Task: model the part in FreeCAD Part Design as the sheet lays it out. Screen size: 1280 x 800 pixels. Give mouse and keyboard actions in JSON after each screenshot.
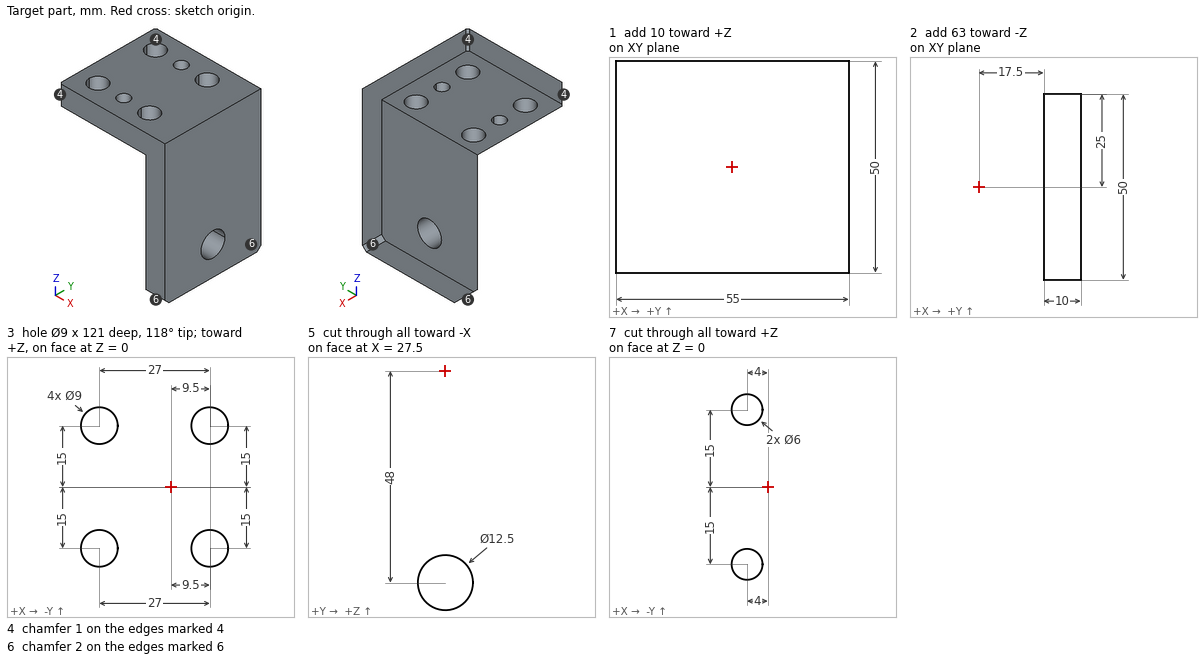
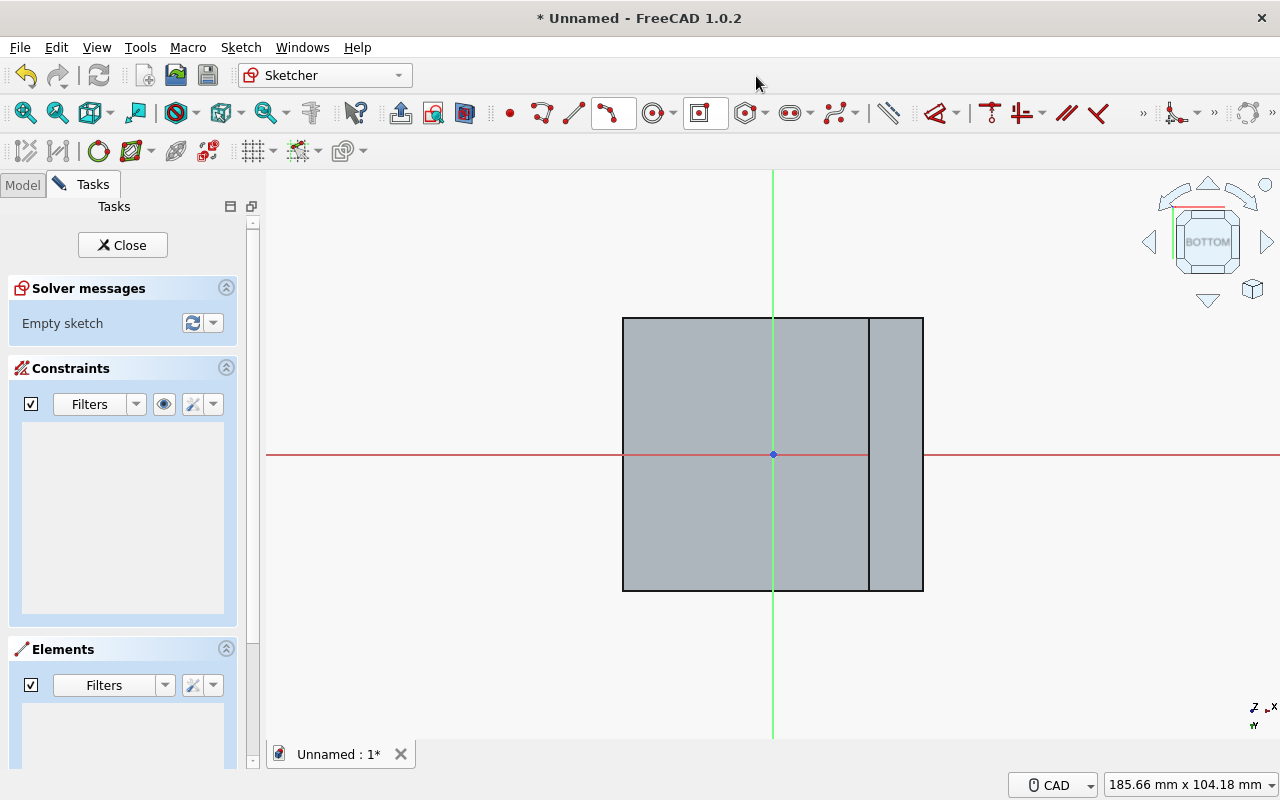
{"action": "left_click", "coordinate": [466, 114]}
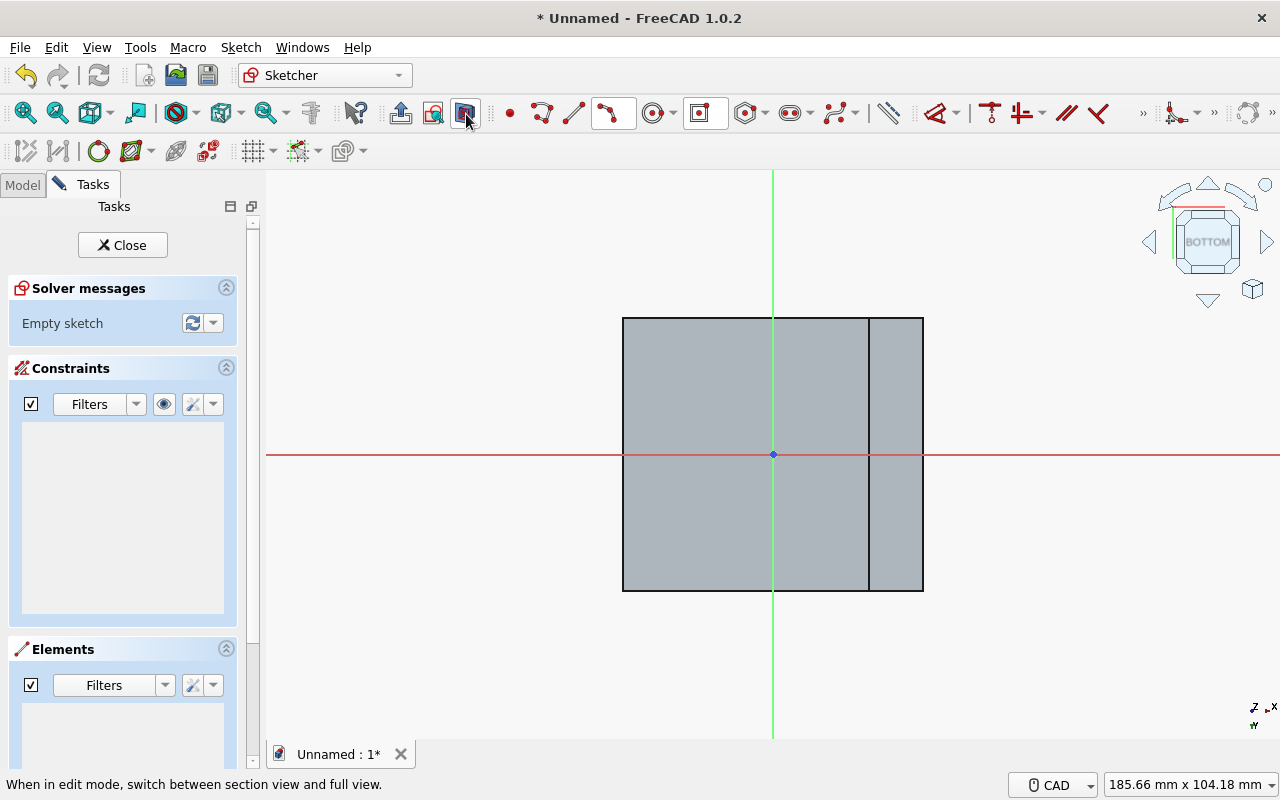
{"action": "scroll", "coordinate": [808, 454], "scroll_direction": "up", "scroll_amount": 3}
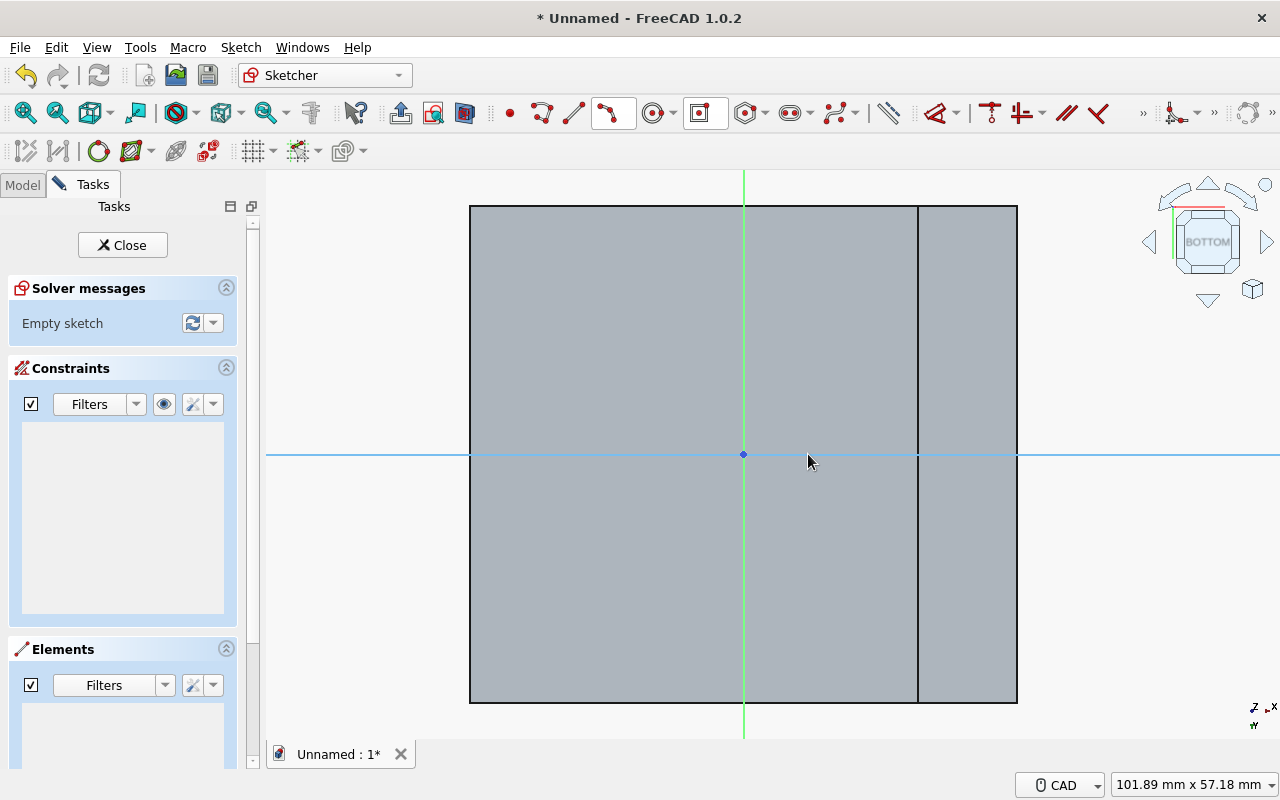
{"action": "key", "text": "g c"}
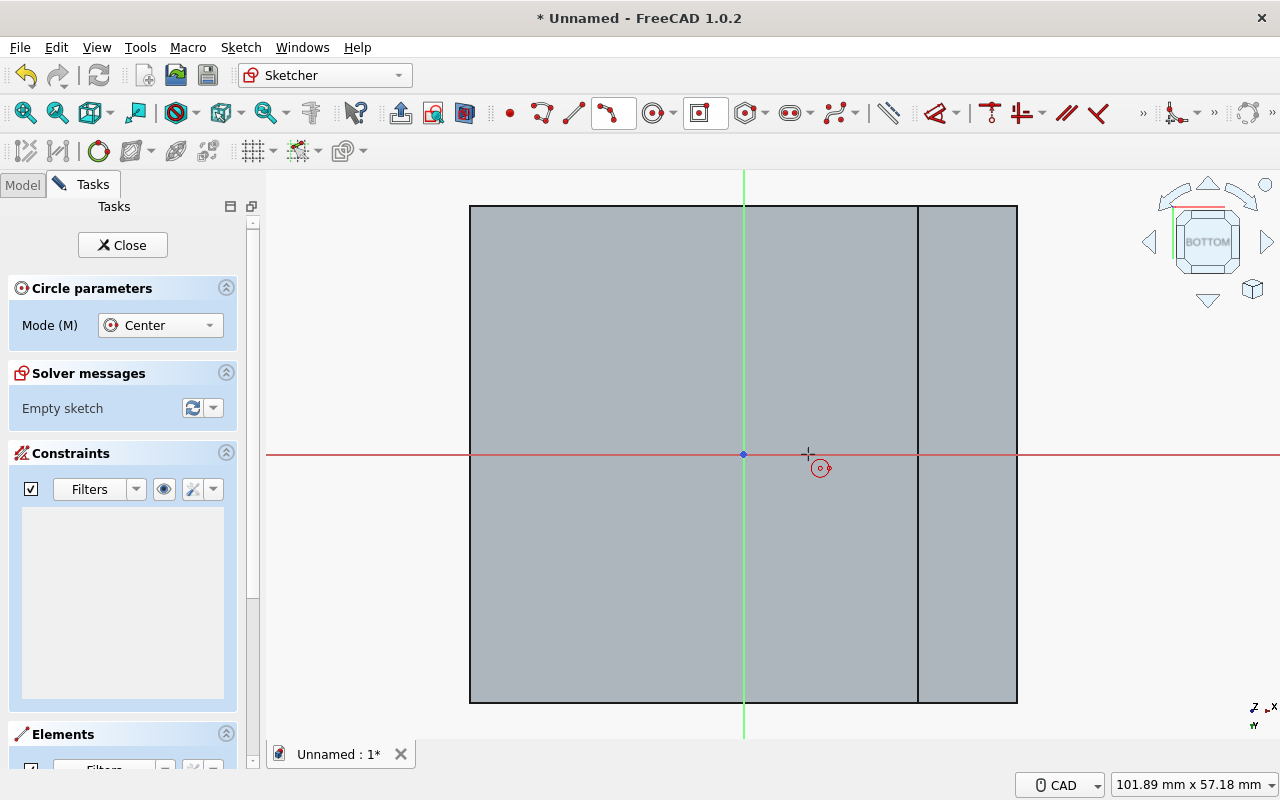
{"action": "left_click", "coordinate": [570, 305]}
{"action": "left_click", "coordinate": [601, 274]}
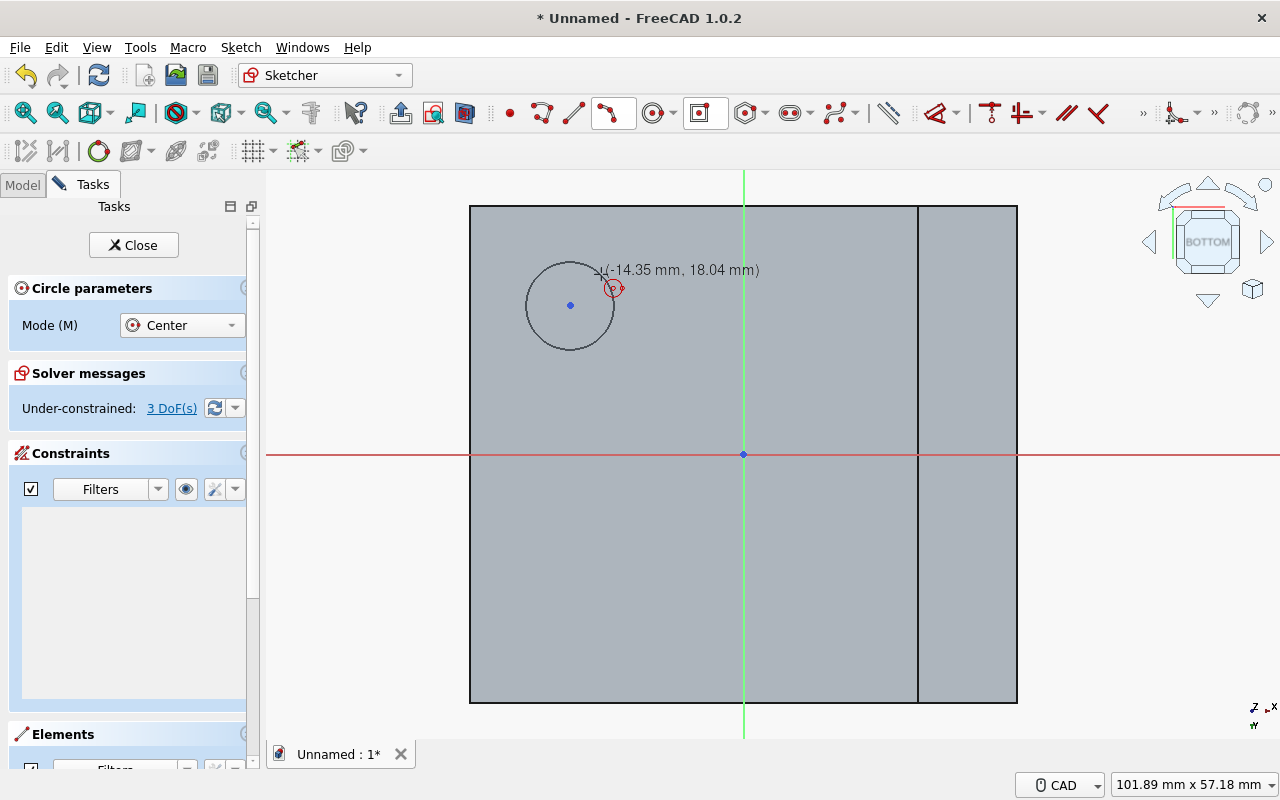
{"action": "left_click", "coordinate": [570, 604]}
{"action": "left_click", "coordinate": [601, 572]}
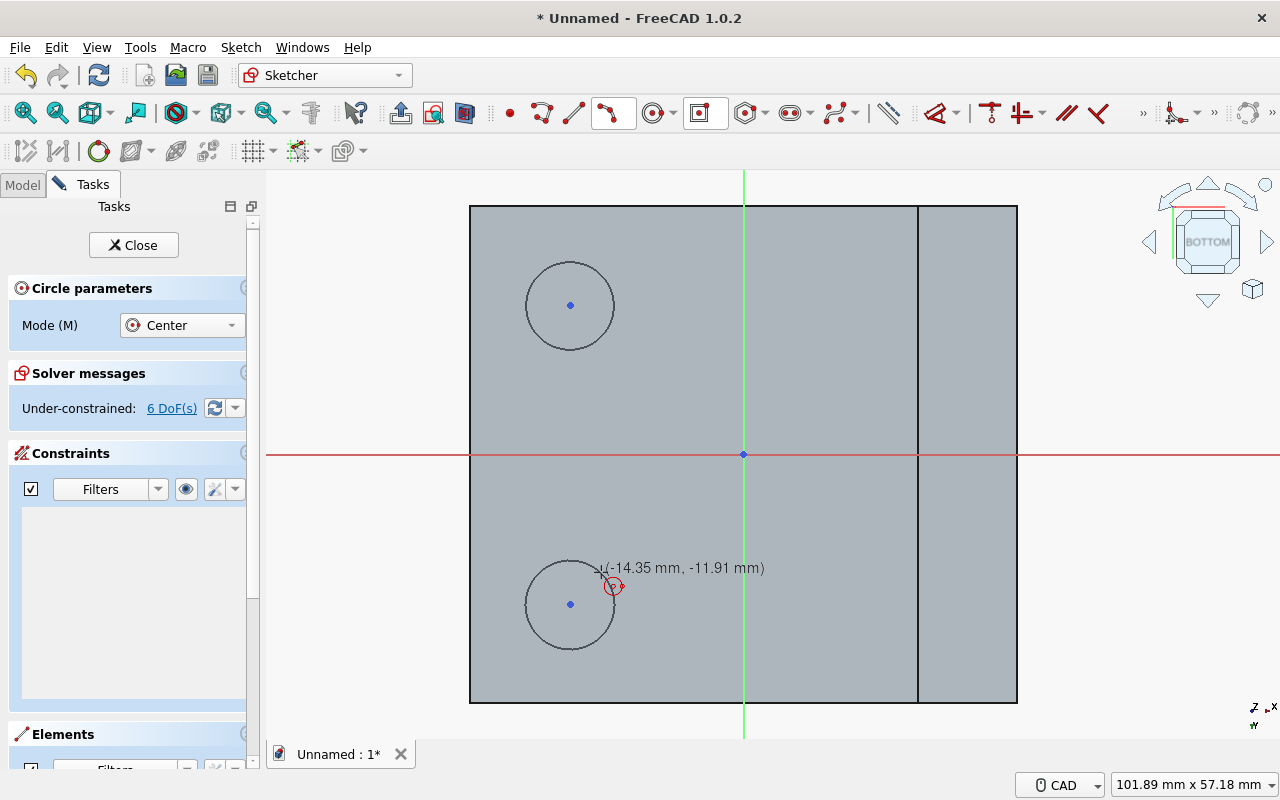
{"action": "left_click", "coordinate": [838, 305]}
{"action": "left_click", "coordinate": [870, 274]}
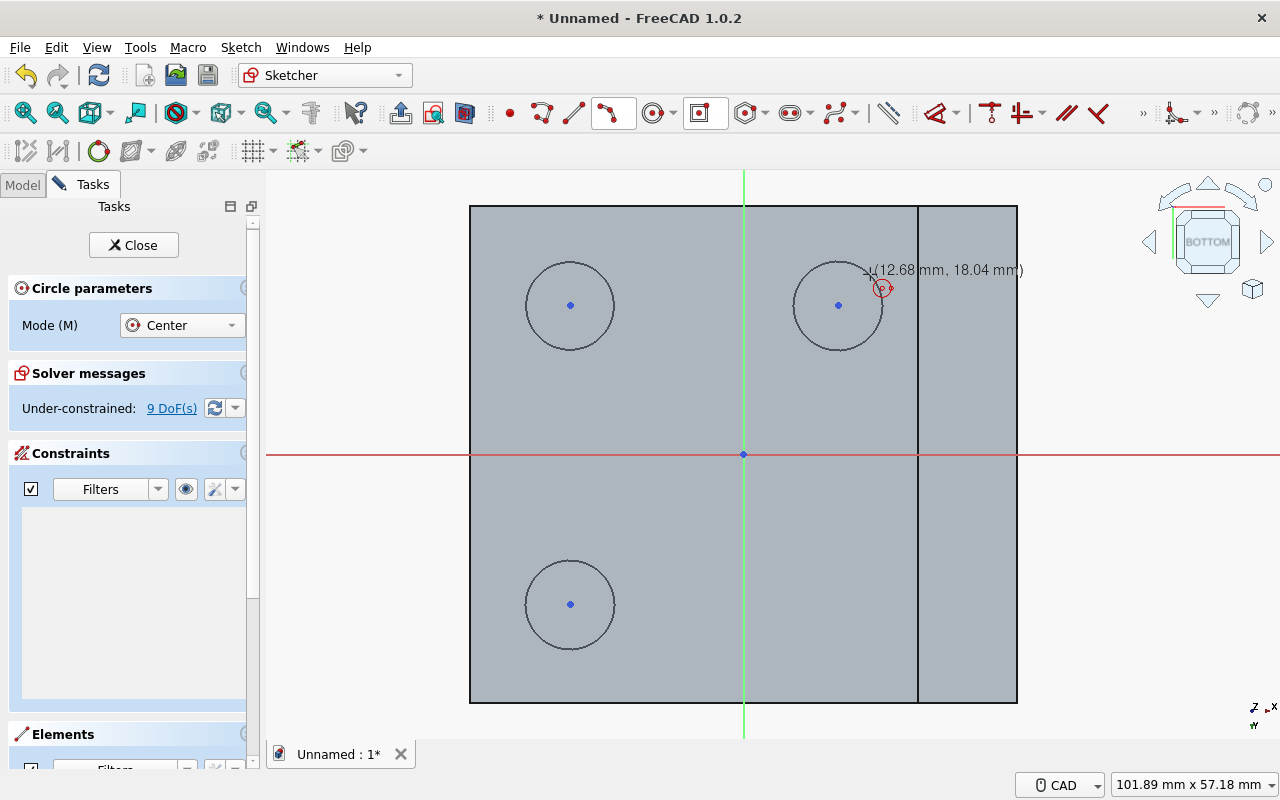
{"action": "left_click", "coordinate": [838, 604]}
{"action": "left_click", "coordinate": [870, 572]}
{"action": "key", "text": "Escape"}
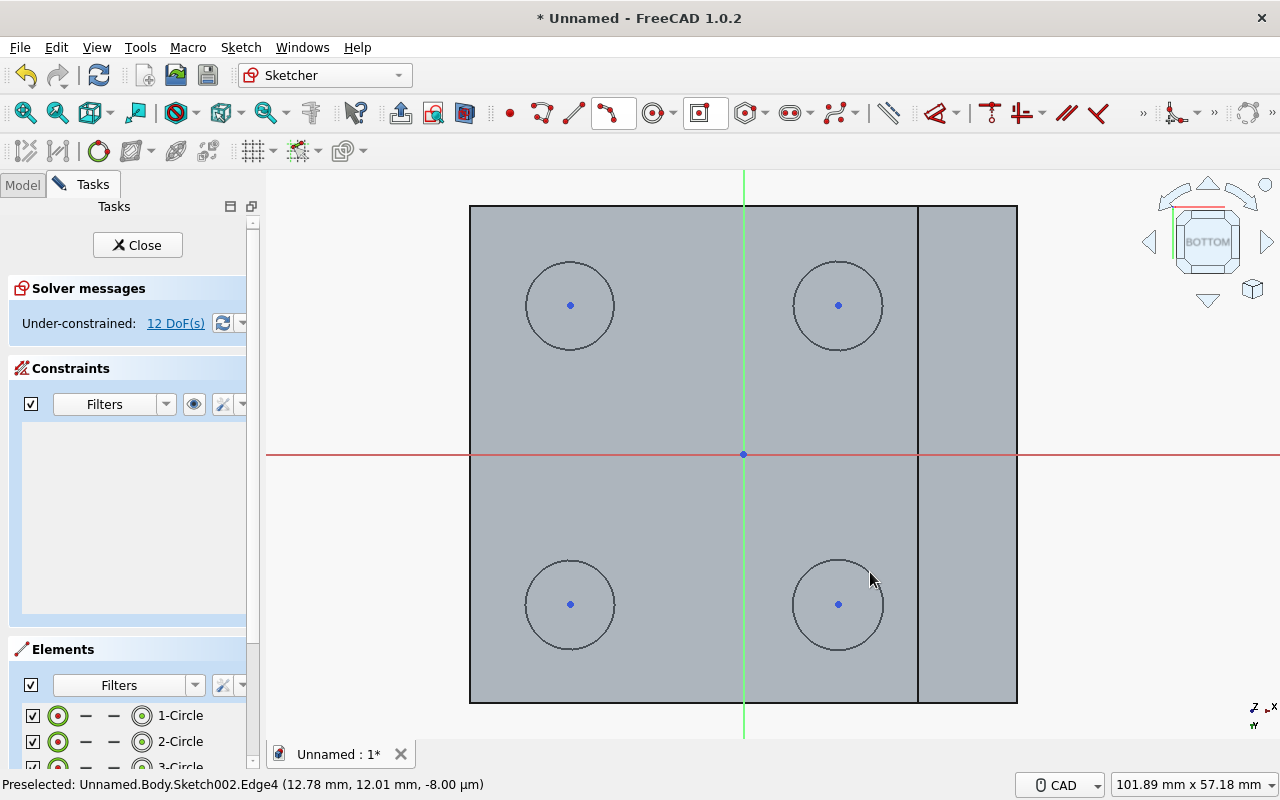
{"action": "left_click", "coordinate": [601, 275]}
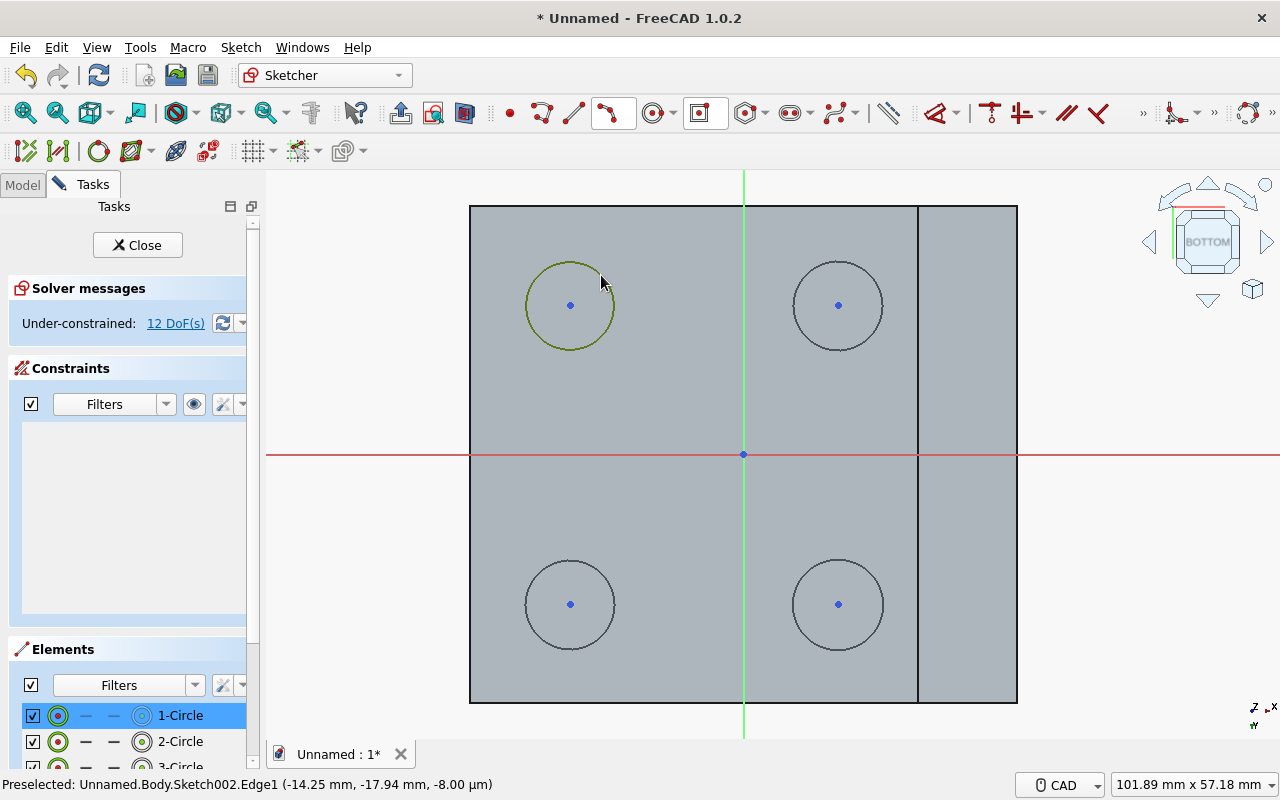
{"action": "left_click", "coordinate": [601, 573]}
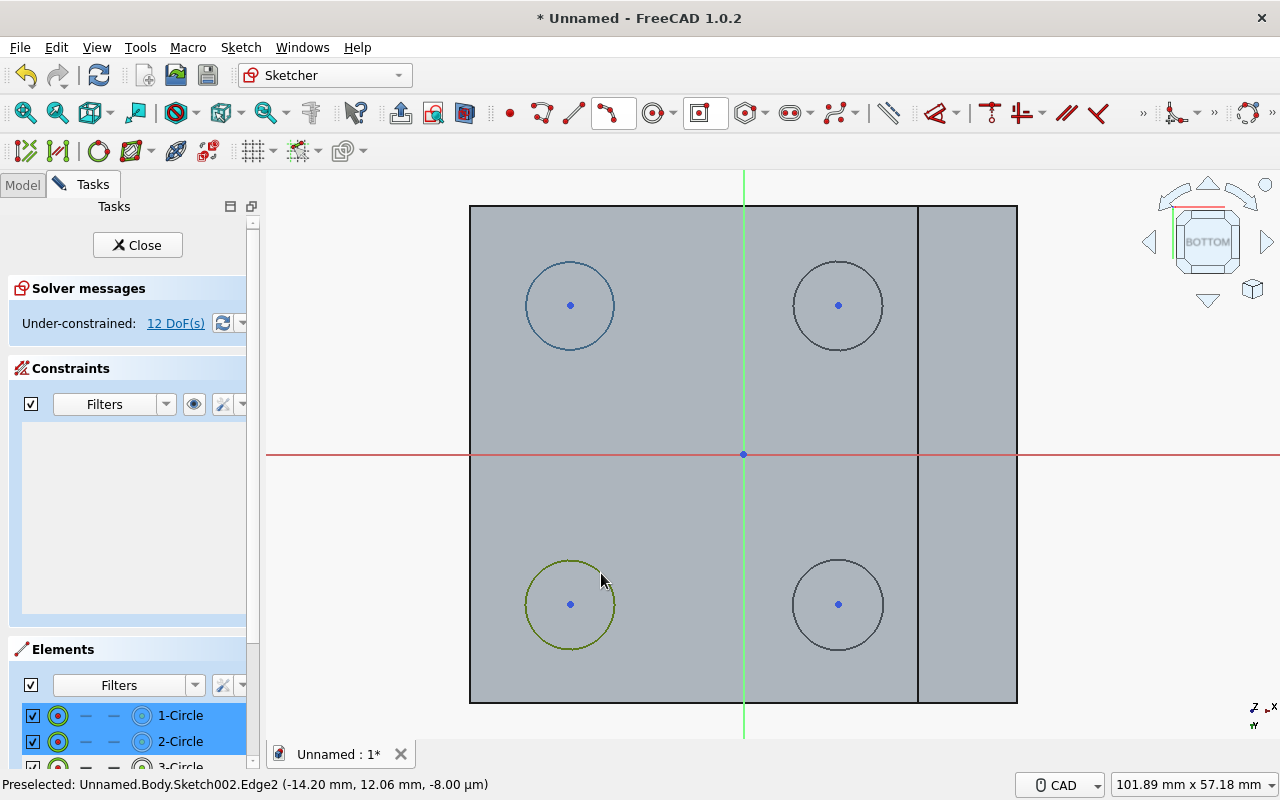
{"action": "left_click", "coordinate": [869, 274]}